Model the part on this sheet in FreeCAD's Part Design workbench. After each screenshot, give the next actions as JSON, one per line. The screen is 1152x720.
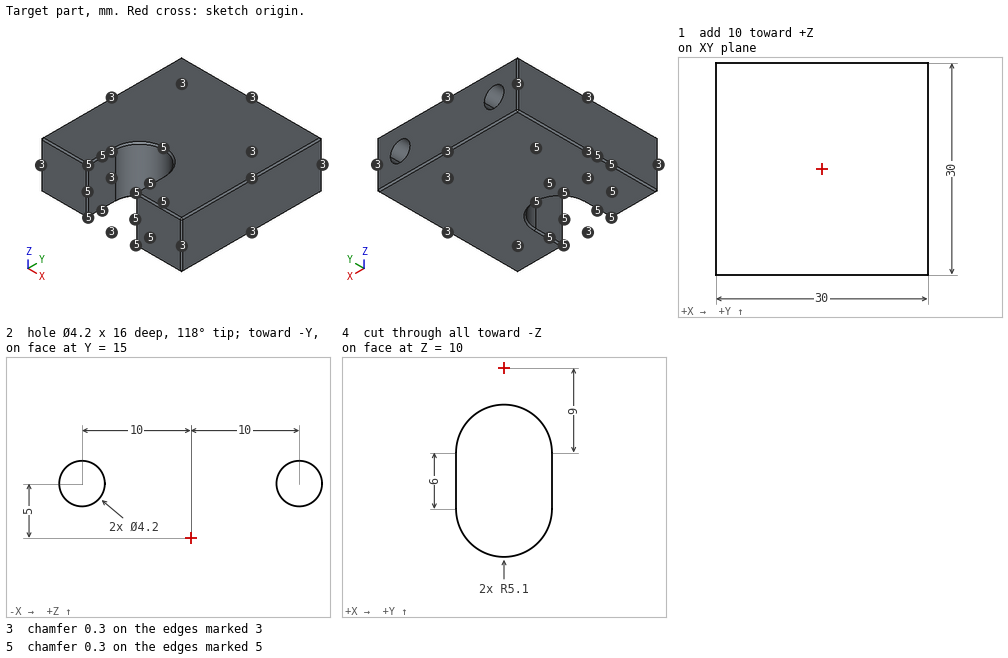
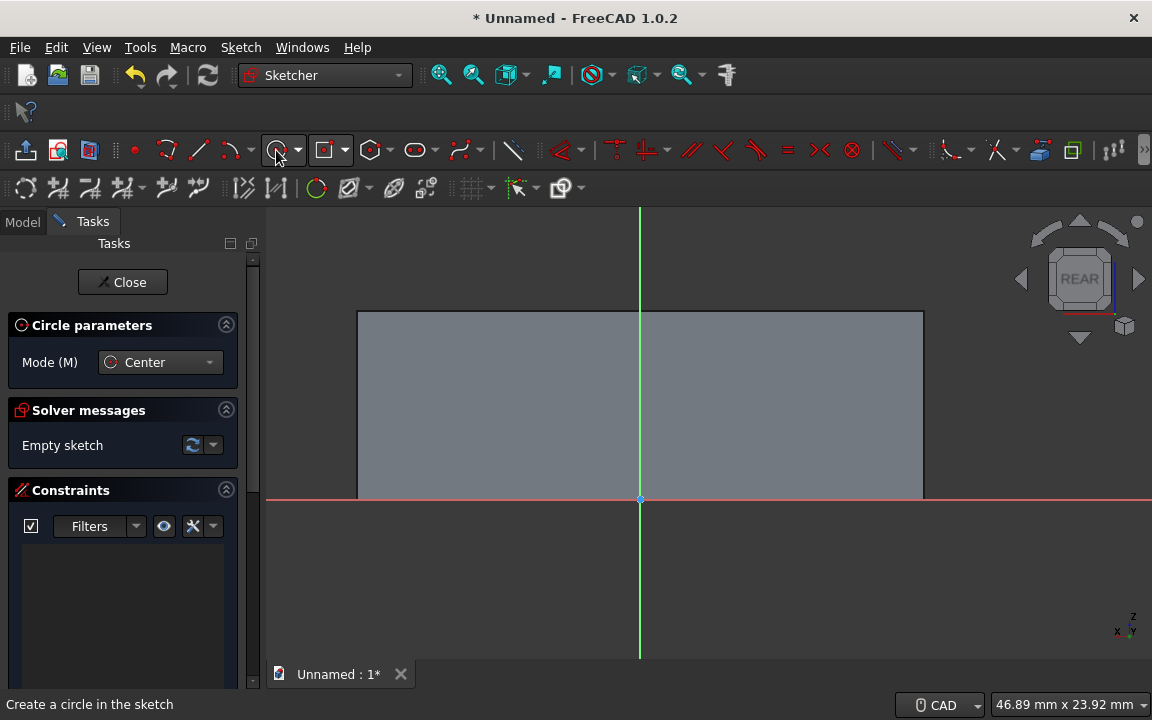
{"action": "left_click", "coordinate": [451, 405]}
{"action": "left_click", "coordinate": [479, 377]}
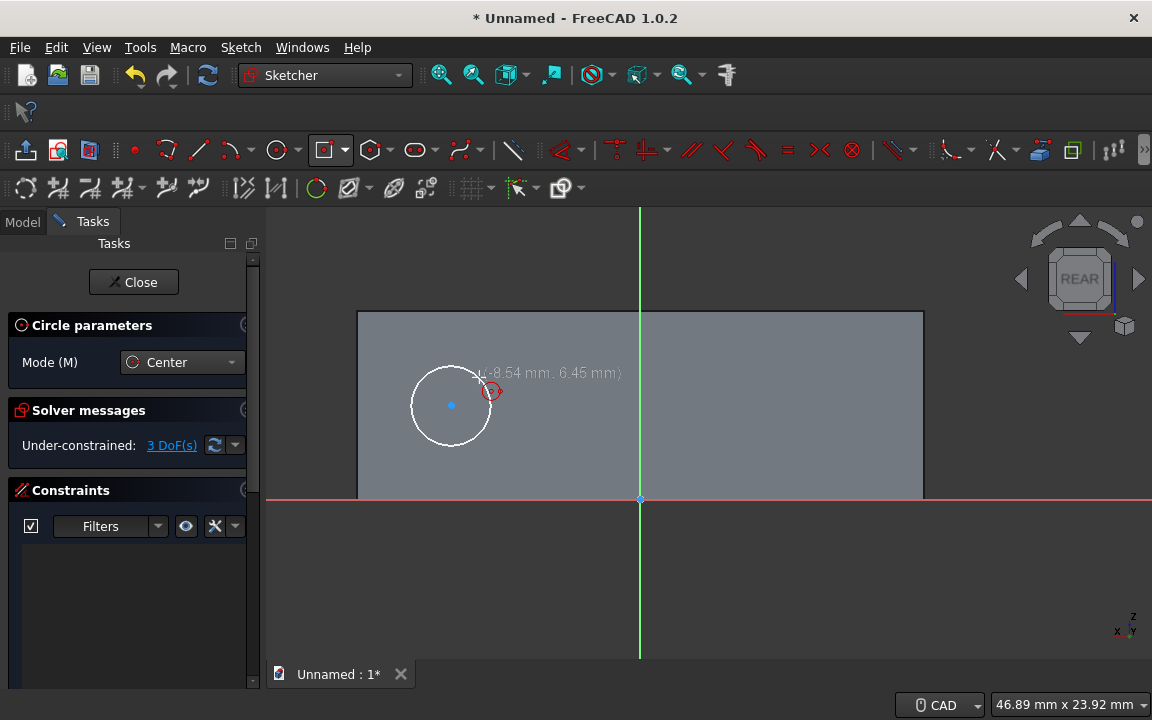
{"action": "left_click", "coordinate": [829, 405]}
{"action": "left_click", "coordinate": [857, 377]}
{"action": "key", "text": "Escape"}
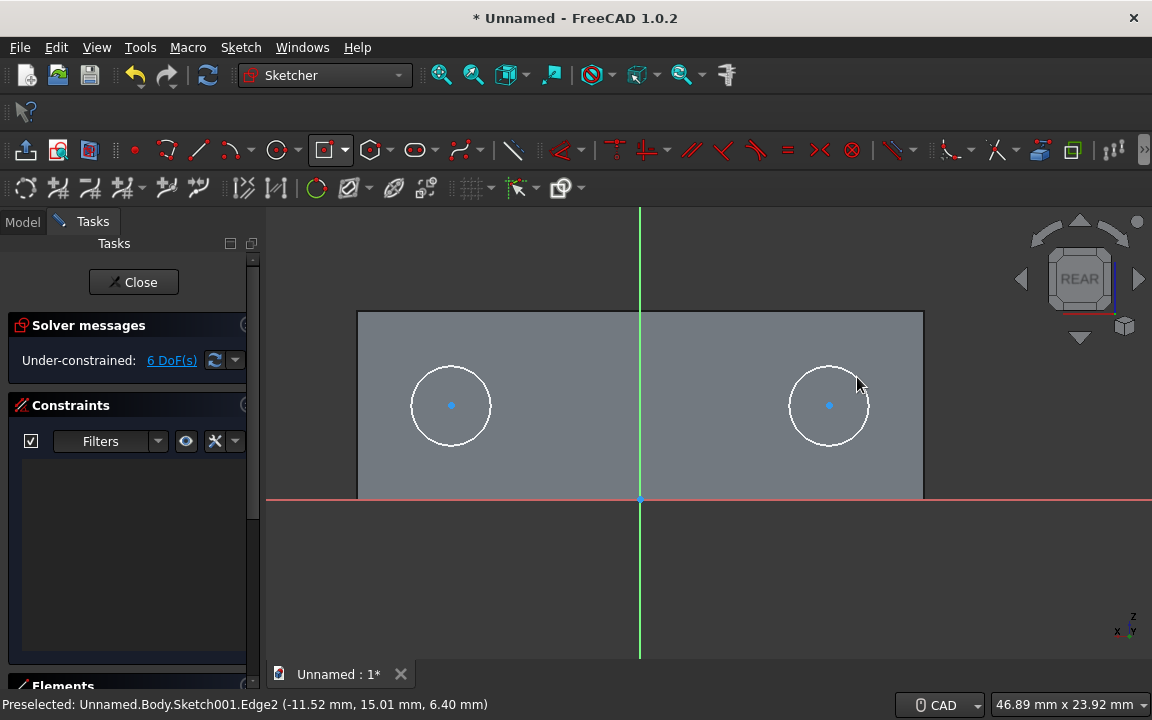
{"action": "left_click", "coordinate": [479, 378]}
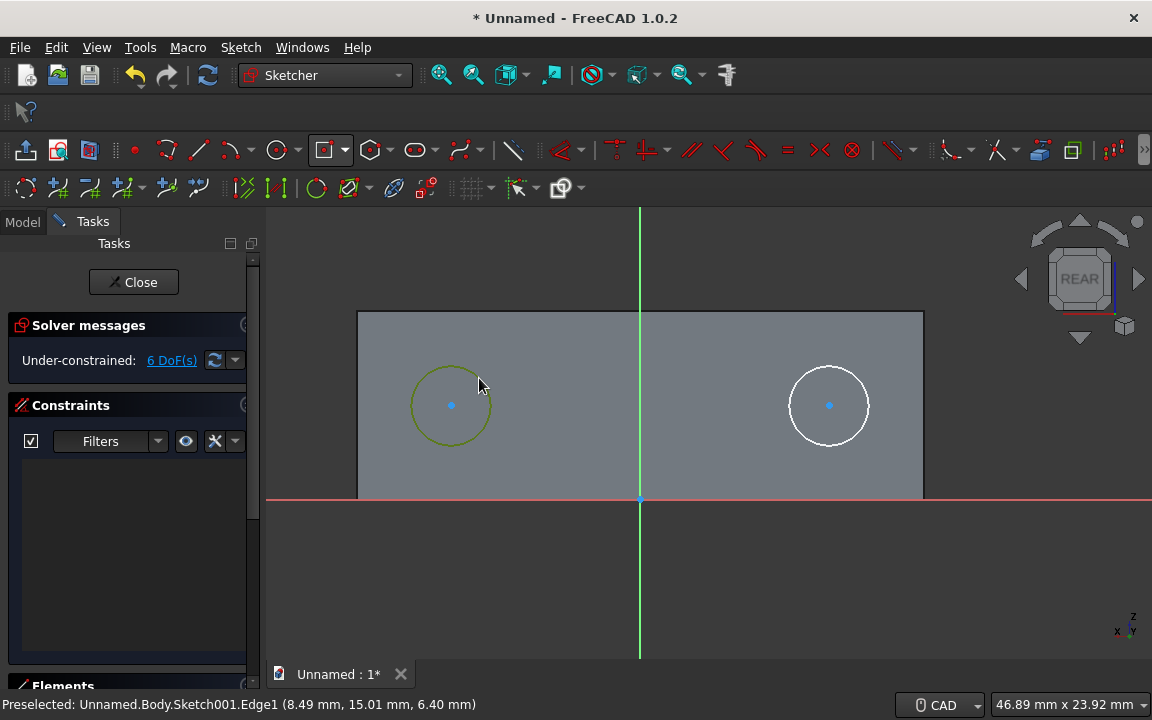
{"action": "left_click", "coordinate": [857, 378]}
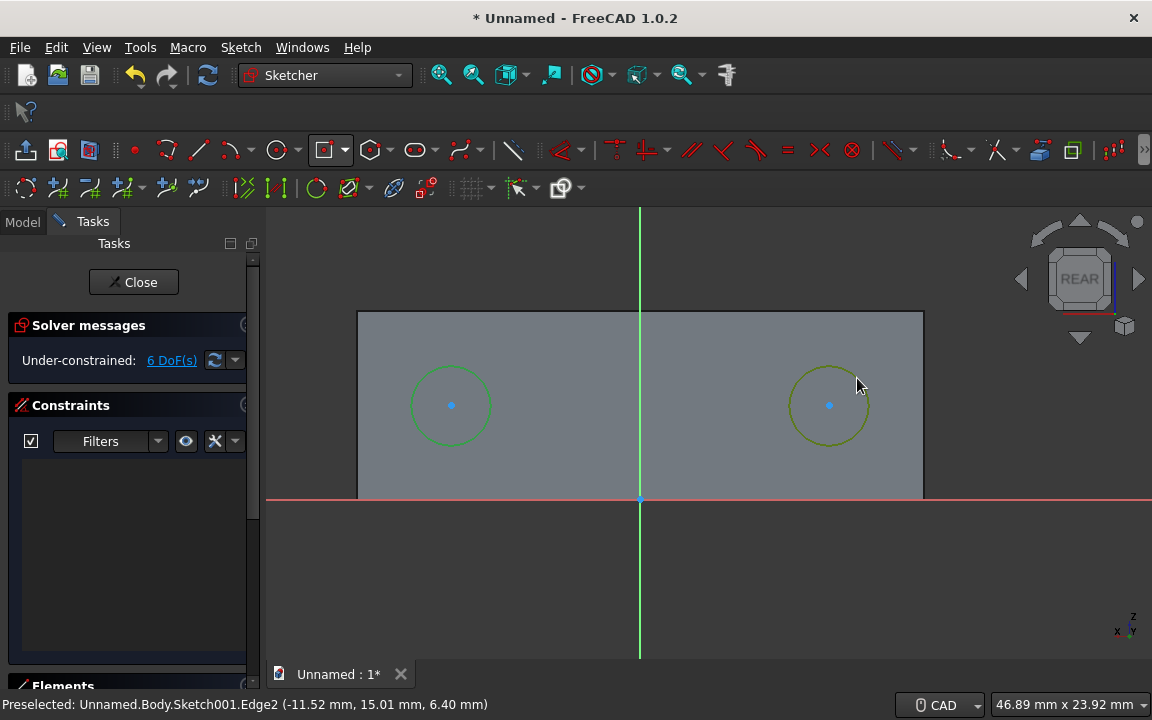
{"action": "left_click", "coordinate": [788, 150]}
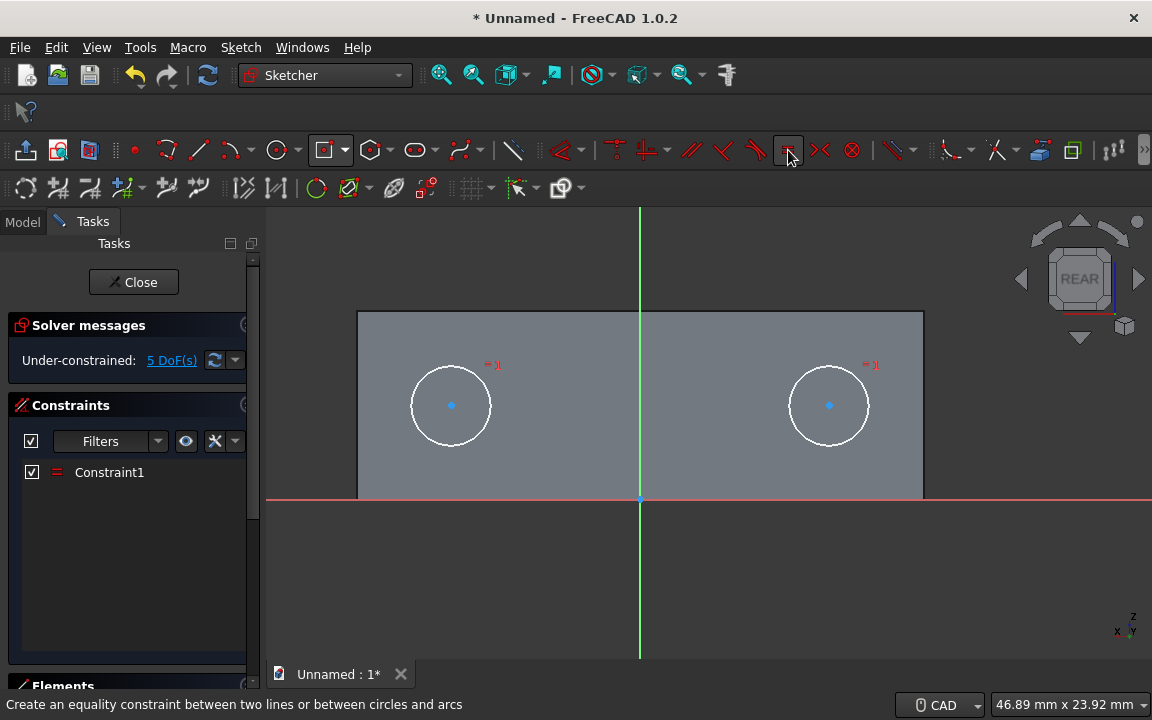
{"action": "left_click", "coordinate": [451, 406]}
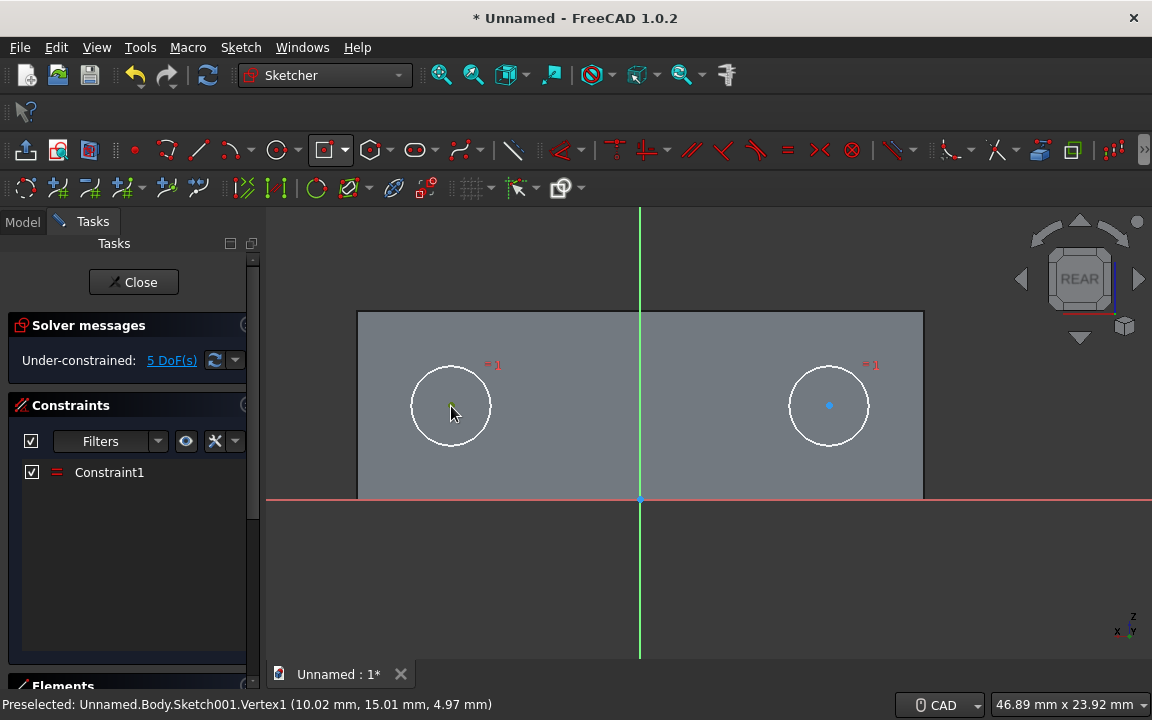
{"action": "left_click", "coordinate": [829, 406]}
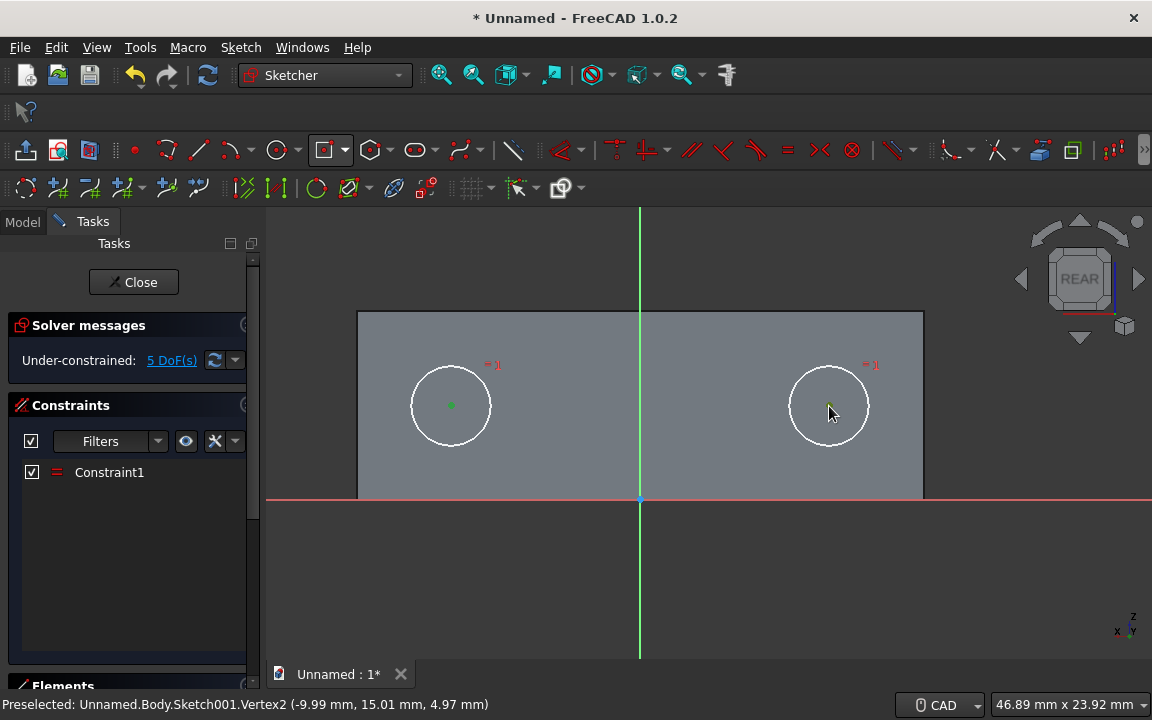
{"action": "left_click", "coordinate": [670, 150]}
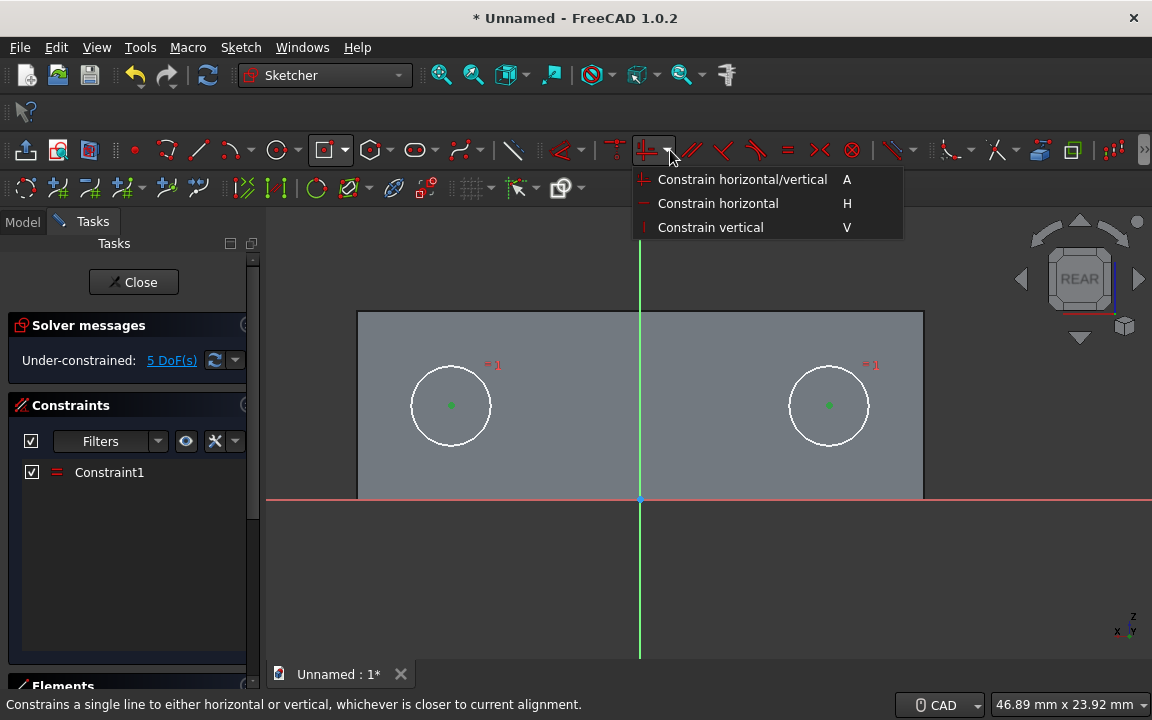
{"action": "left_click", "coordinate": [768, 203]}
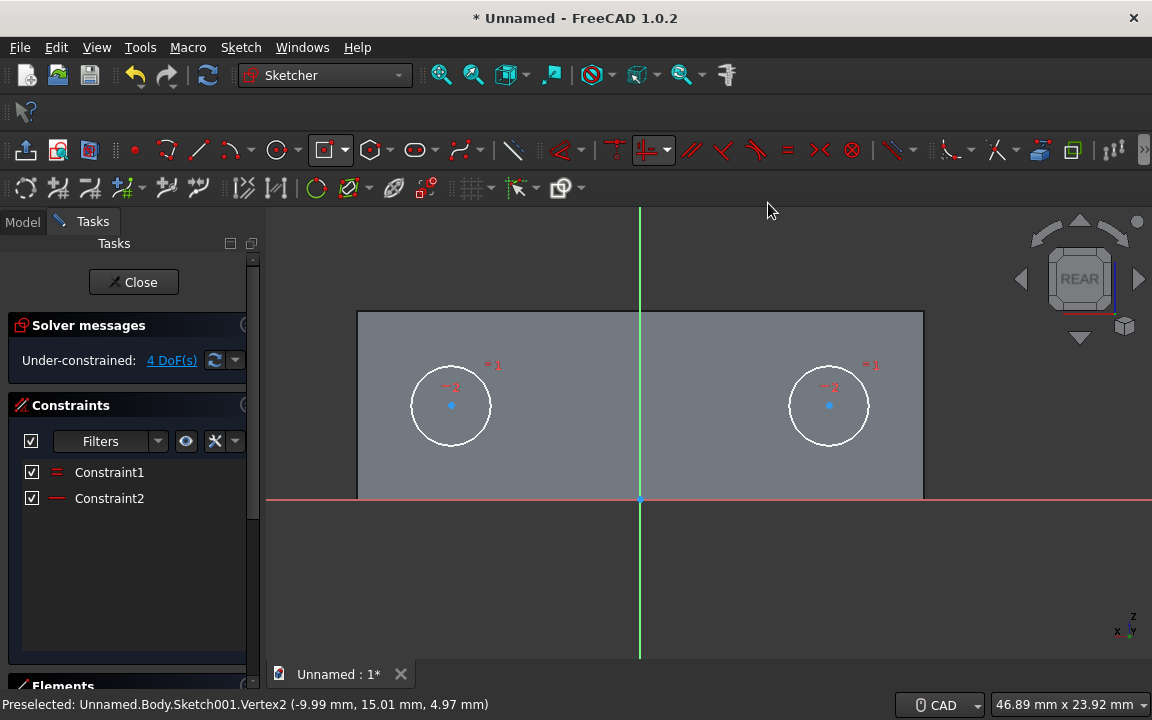
{"action": "left_click", "coordinate": [560, 150]}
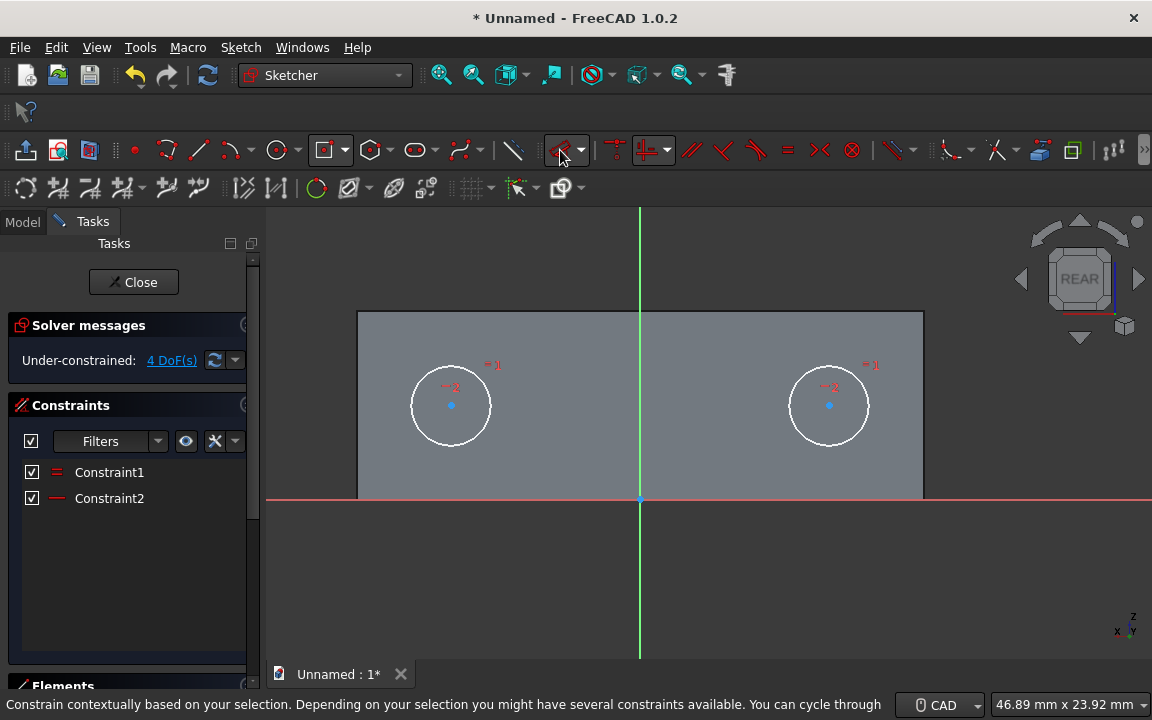
{"action": "left_click", "coordinate": [479, 378]}
{"action": "left_click", "coordinate": [502, 355]}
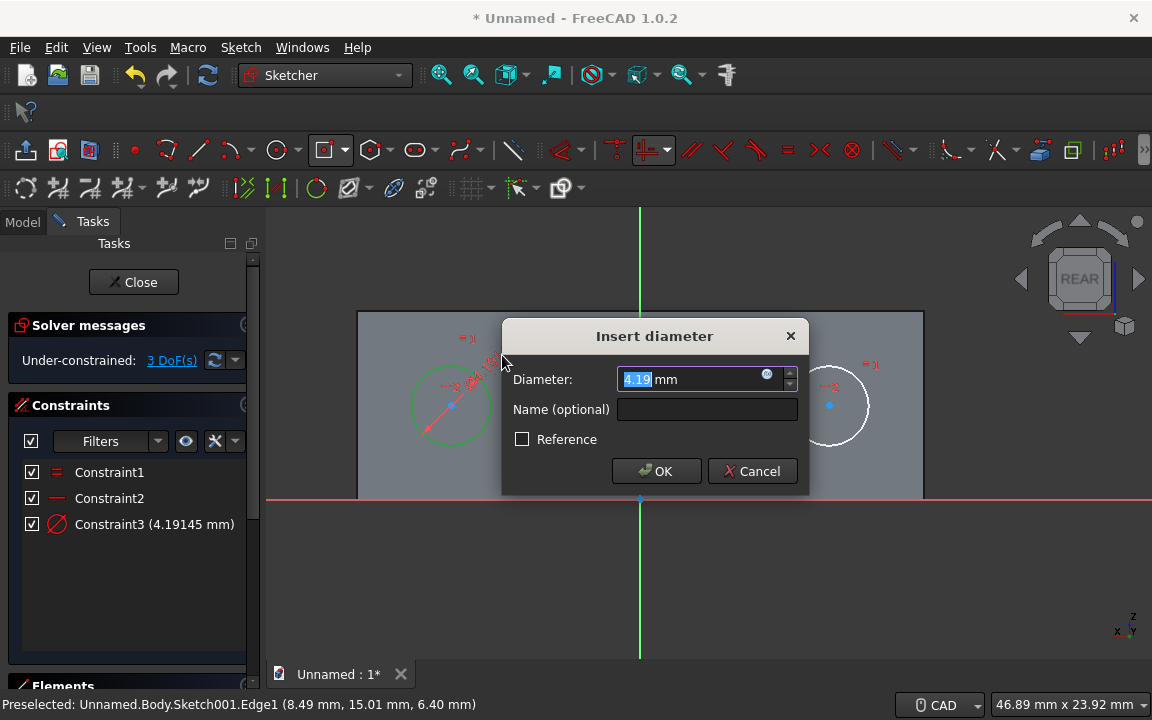
{"action": "type", "text": "4.2"}
{"action": "key", "text": "Return"}